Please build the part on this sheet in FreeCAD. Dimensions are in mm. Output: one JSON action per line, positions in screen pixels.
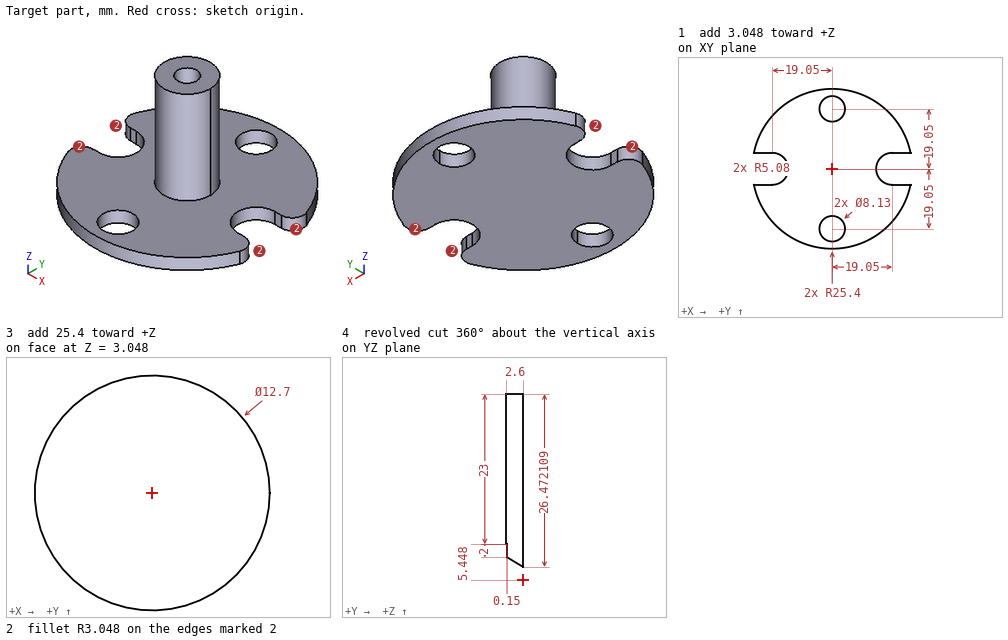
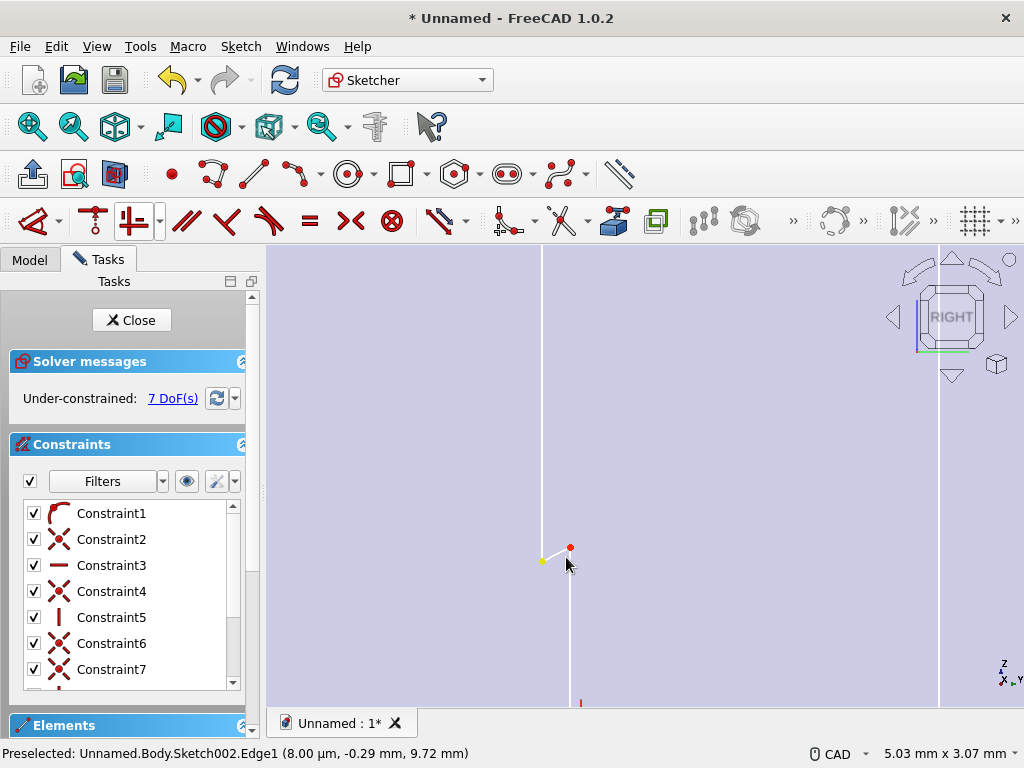
{"action": "left_click", "coordinate": [556, 554]}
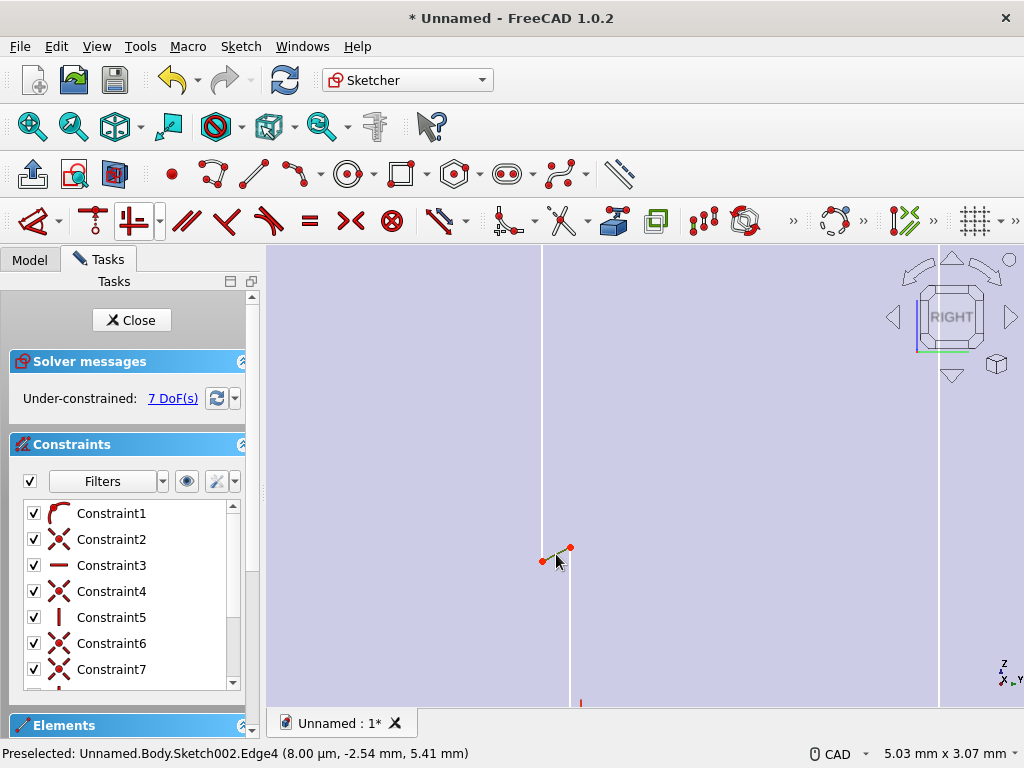
{"action": "left_click", "coordinate": [160, 222]}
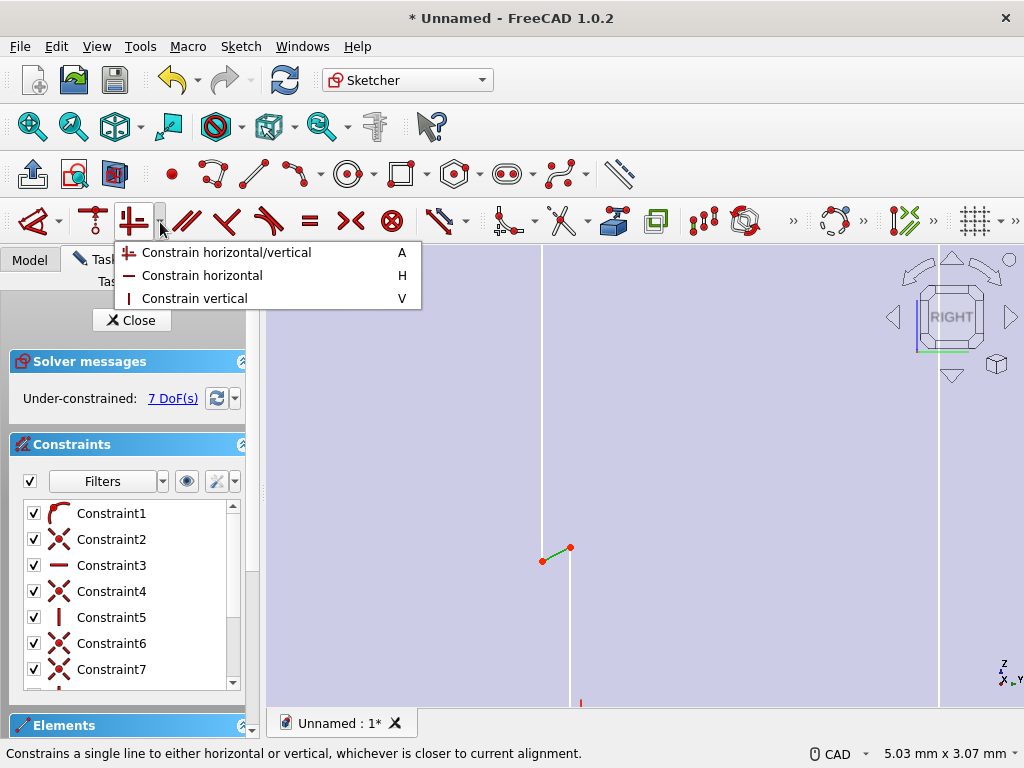
{"action": "left_click", "coordinate": [268, 276]}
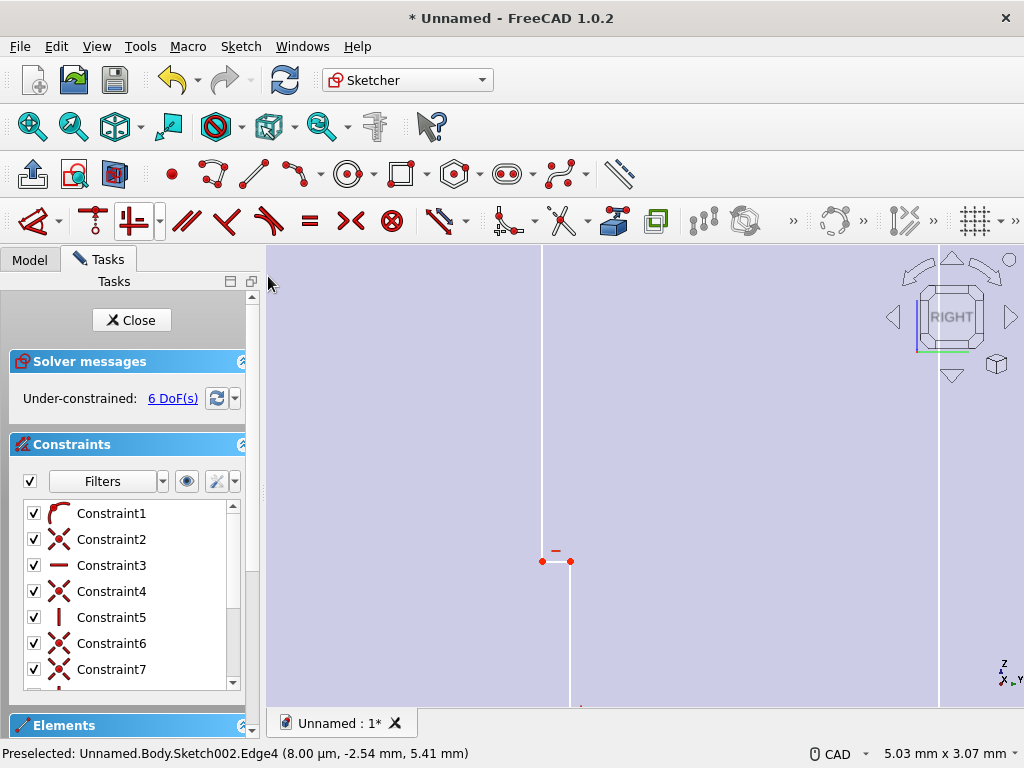
{"action": "left_click", "coordinate": [32, 222]}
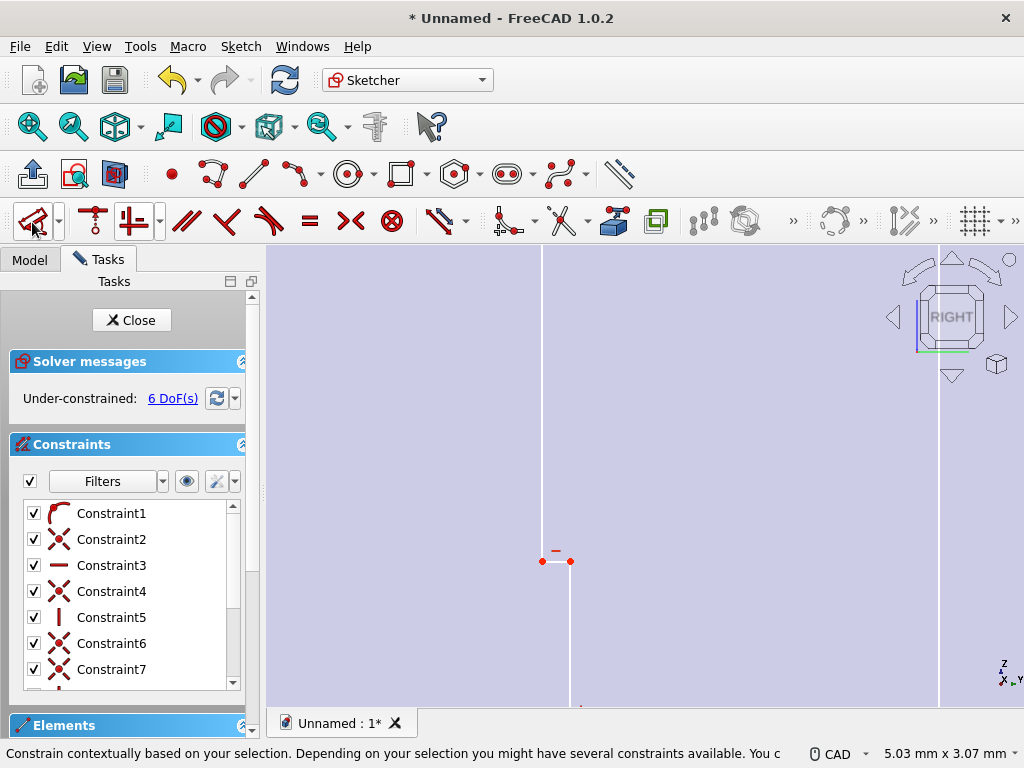
{"action": "scroll", "coordinate": [566, 557], "scroll_direction": "down", "scroll_amount": 14}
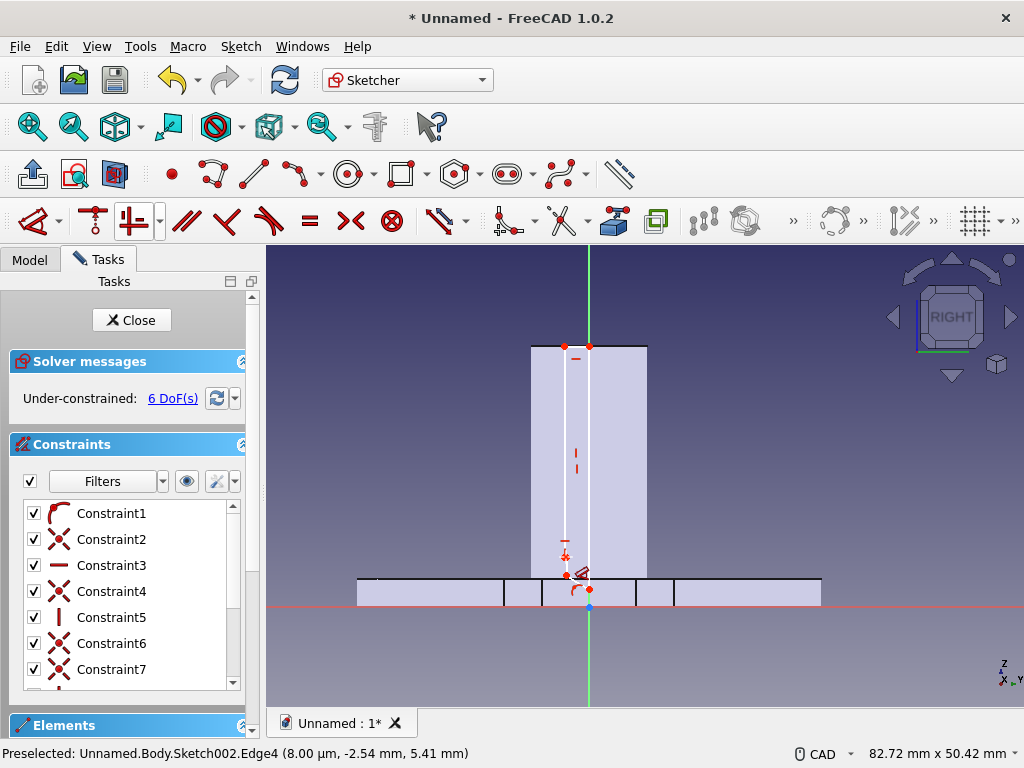
{"action": "scroll", "coordinate": [567, 563], "scroll_direction": "up", "scroll_amount": 5}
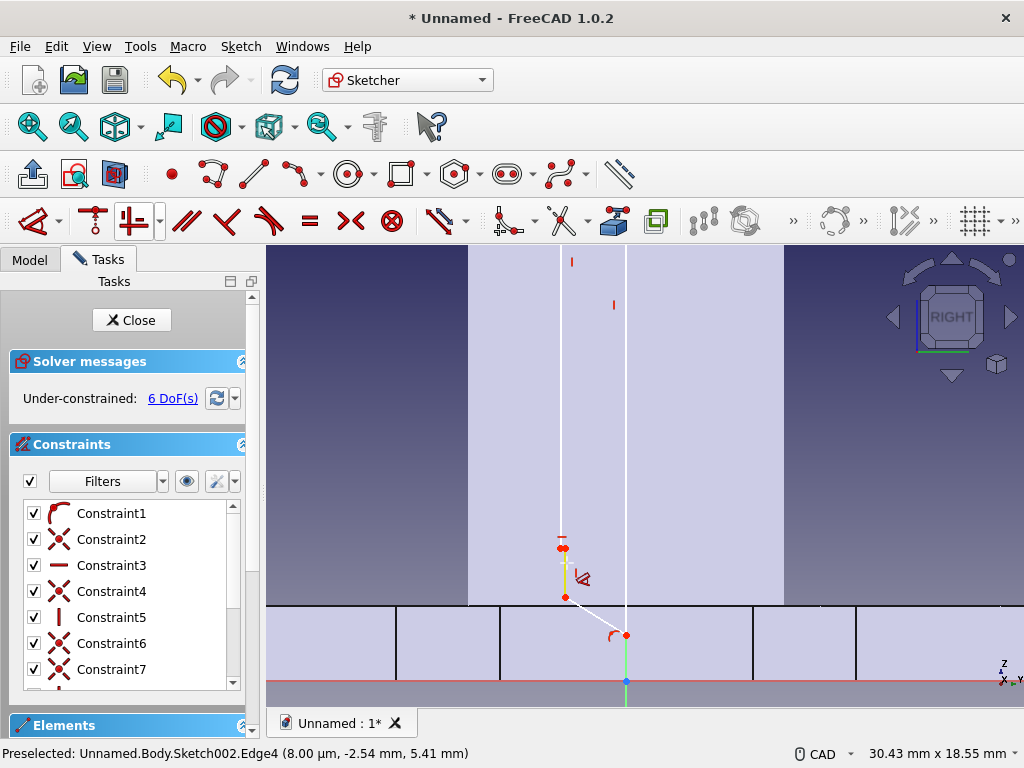
{"action": "left_click", "coordinate": [565, 563]}
{"action": "left_click", "coordinate": [531, 573]}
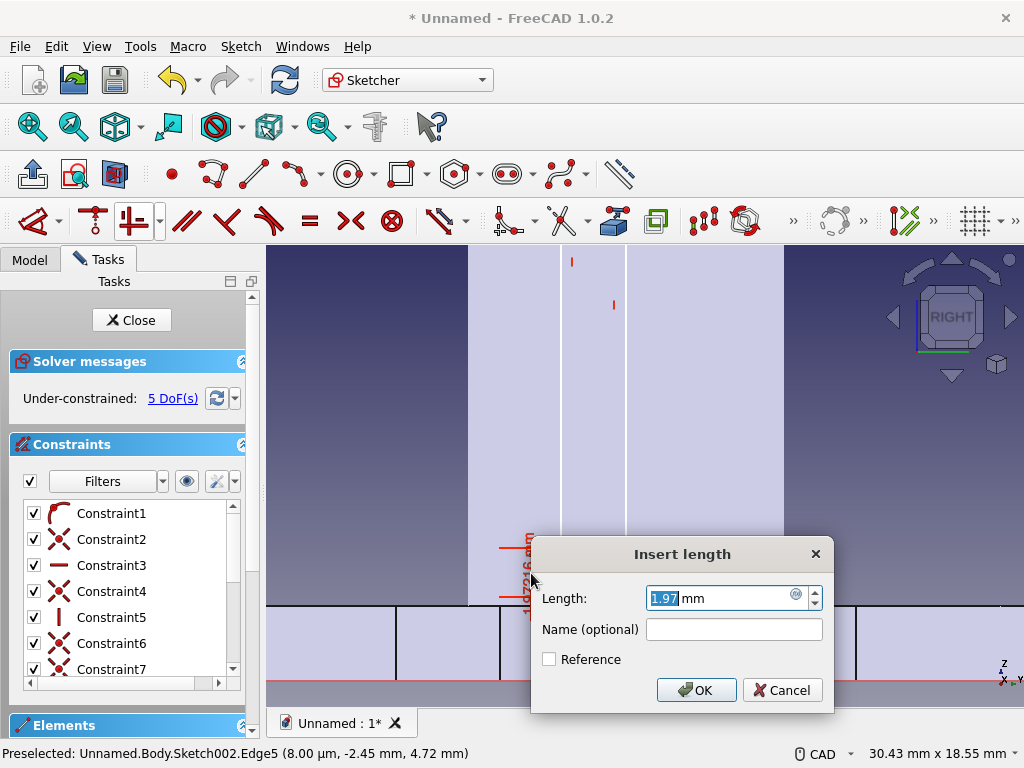
{"action": "type", "text": "2"}
{"action": "key", "text": "Return"}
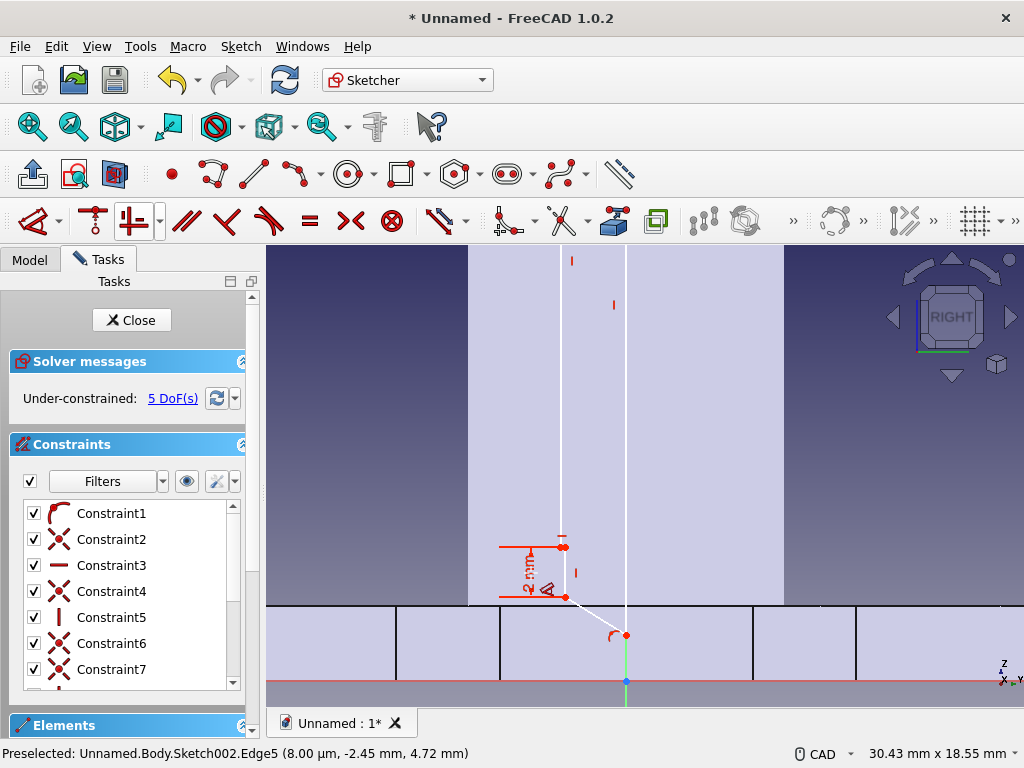
{"action": "left_click", "coordinate": [561, 375]}
{"action": "left_click", "coordinate": [527, 410]}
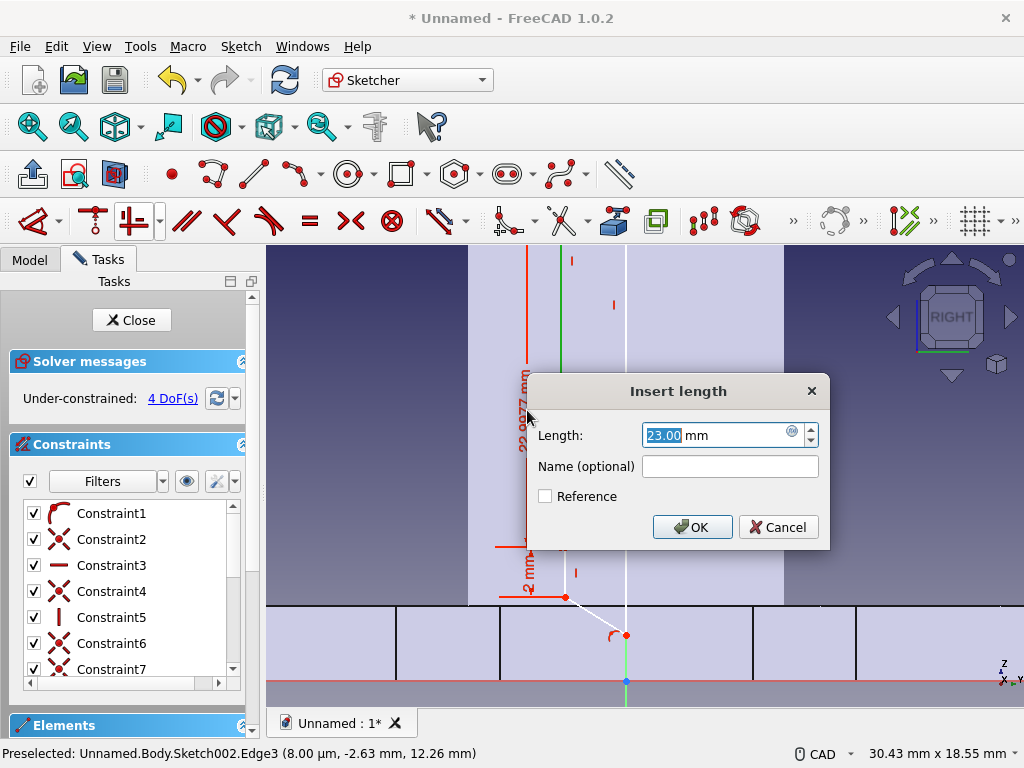
{"action": "type", "text": "23"}
{"action": "key", "text": "Return"}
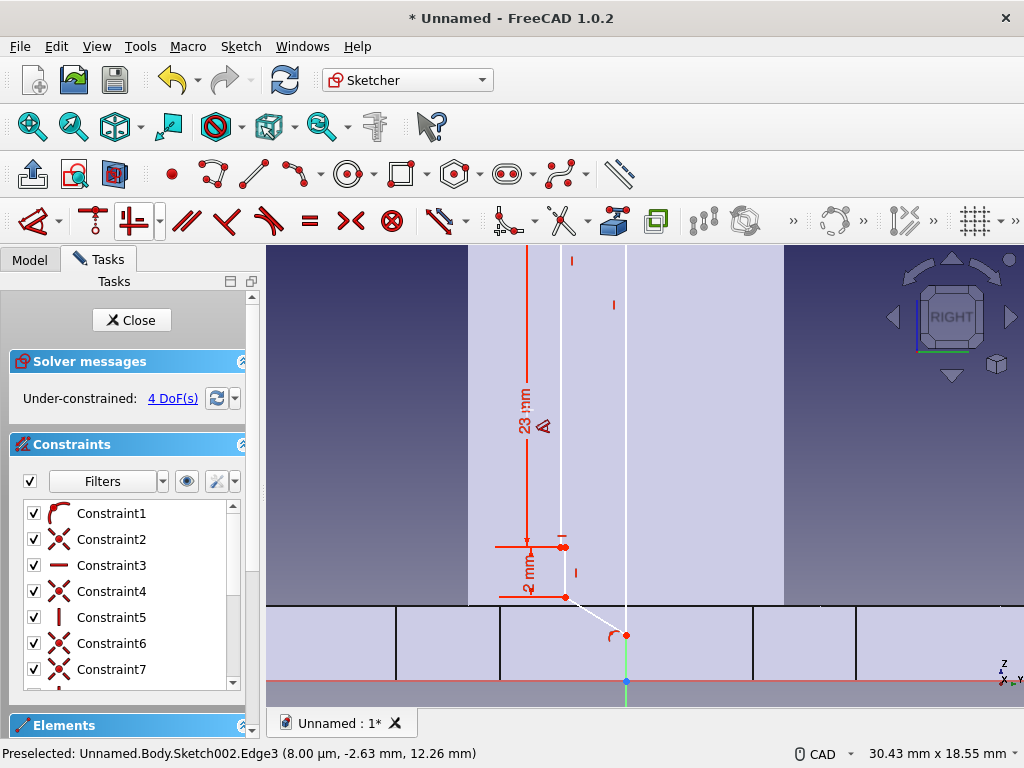
{"action": "scroll", "coordinate": [566, 563], "scroll_direction": "down", "scroll_amount": 5}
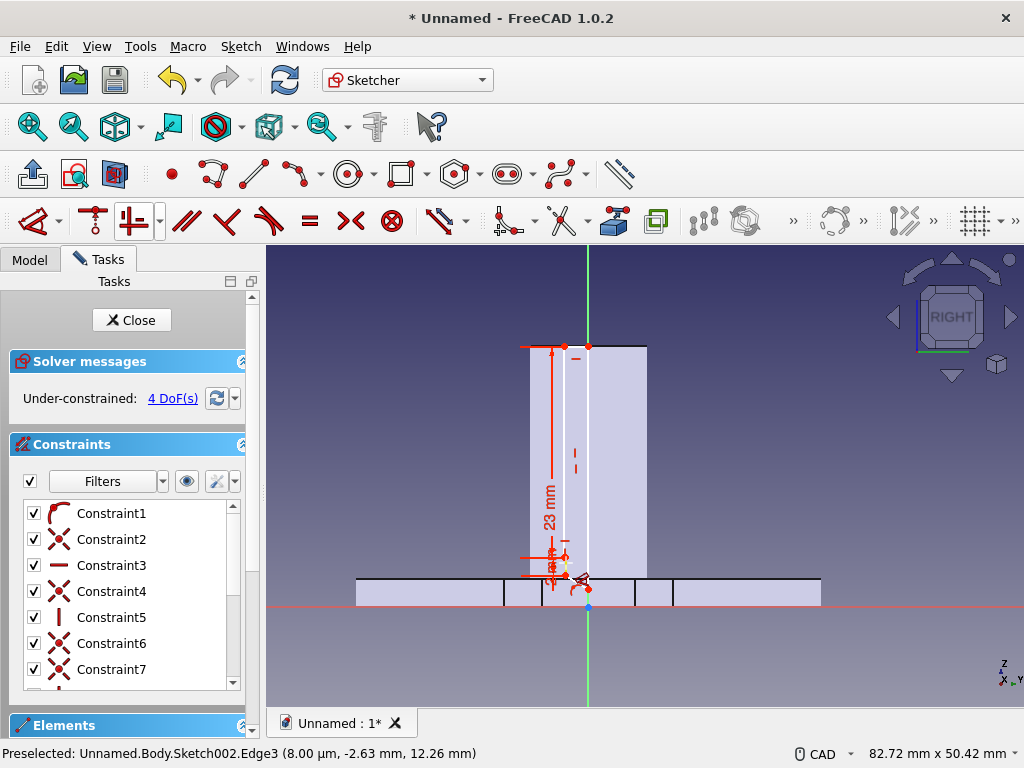
{"action": "scroll", "coordinate": [581, 347], "scroll_direction": "up", "scroll_amount": 4}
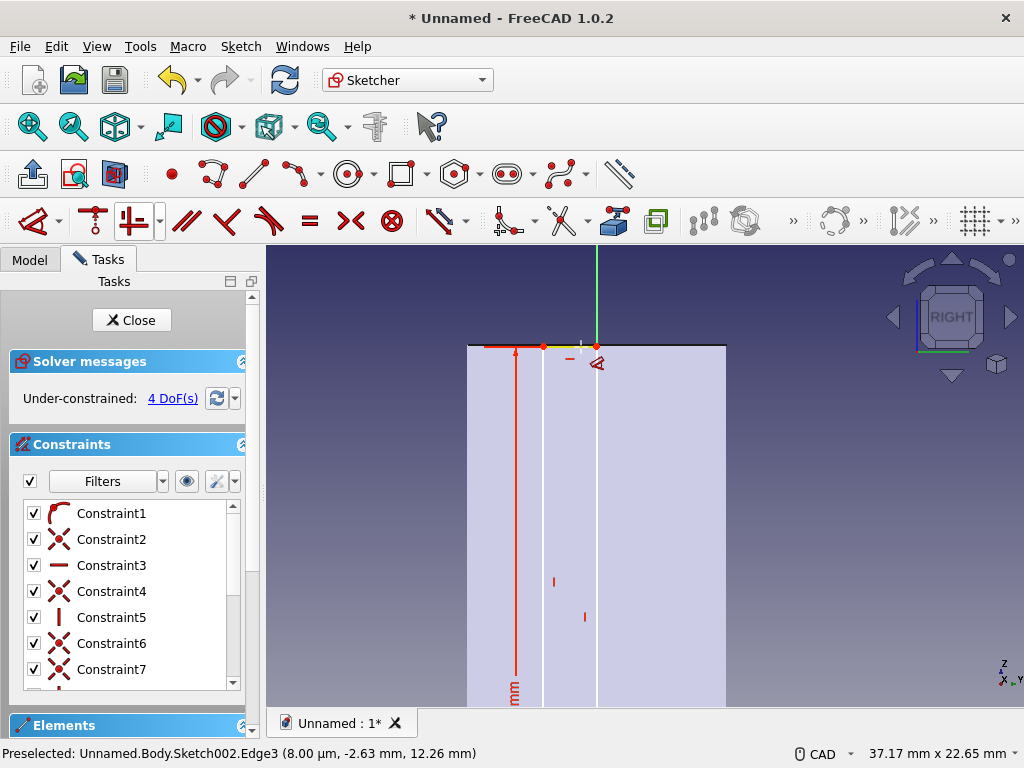
{"action": "left_click", "coordinate": [581, 347]}
{"action": "left_click", "coordinate": [570, 313]}